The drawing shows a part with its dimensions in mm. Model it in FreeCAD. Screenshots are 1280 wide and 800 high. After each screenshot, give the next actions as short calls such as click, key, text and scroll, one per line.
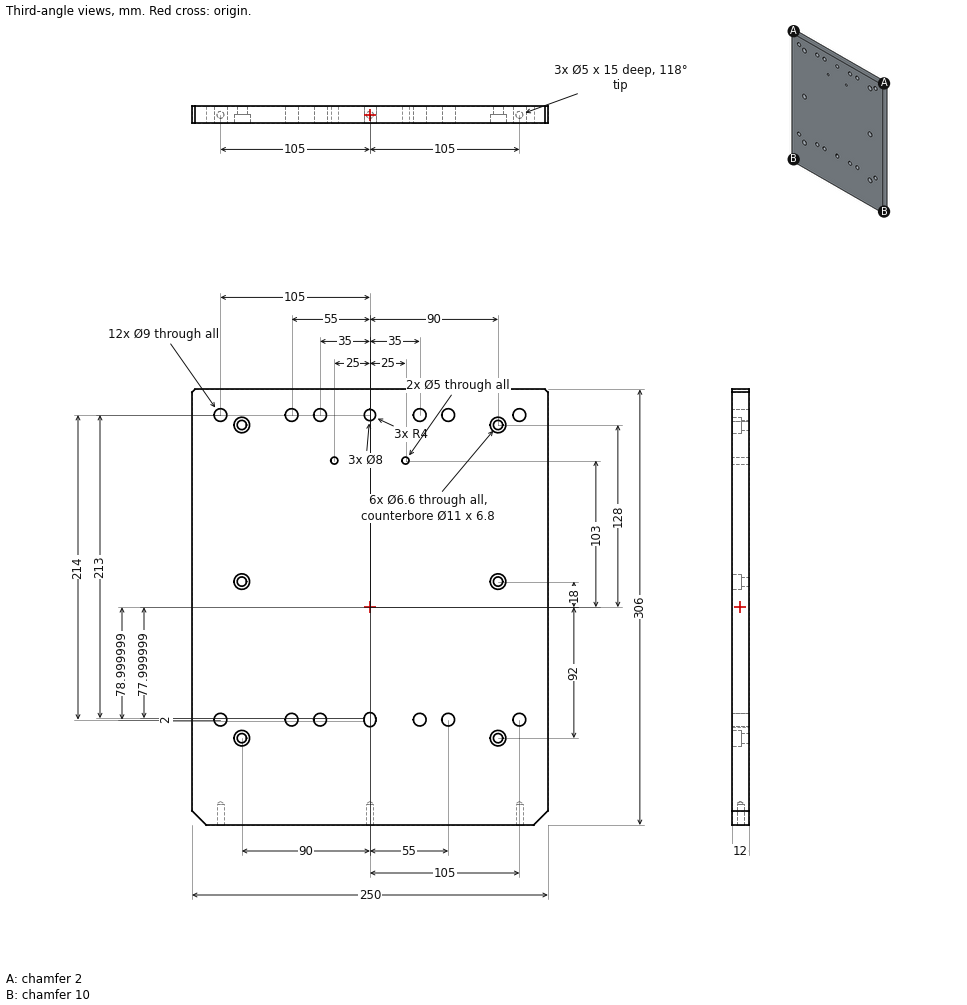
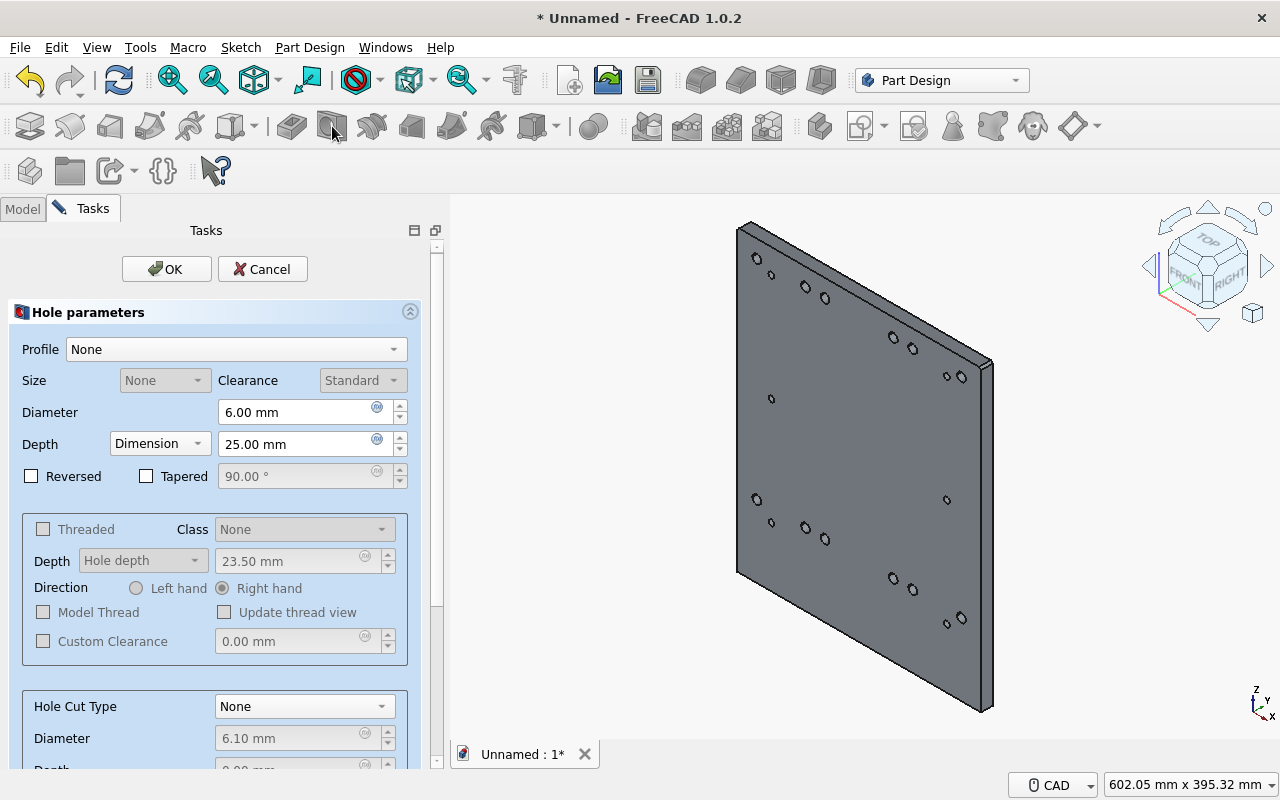
triple_click(305, 412)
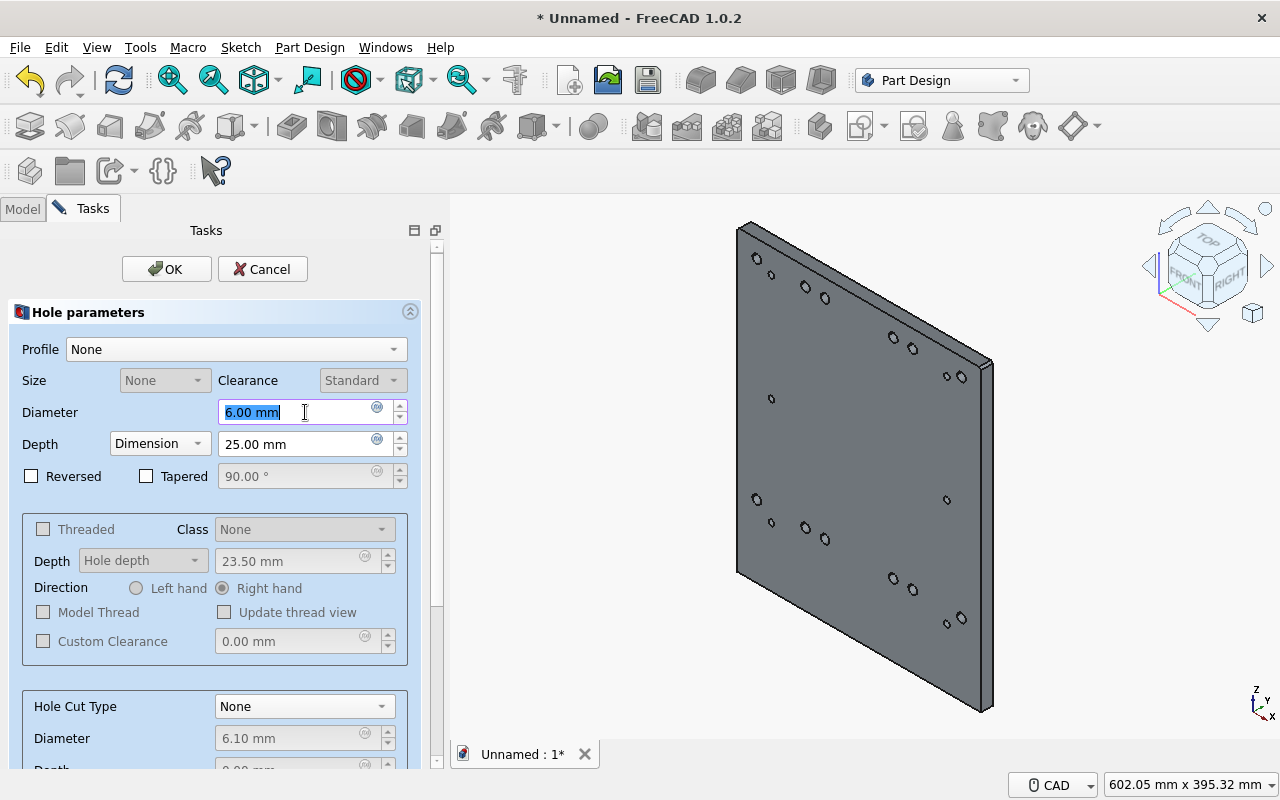
text(6.6)
key(Tab)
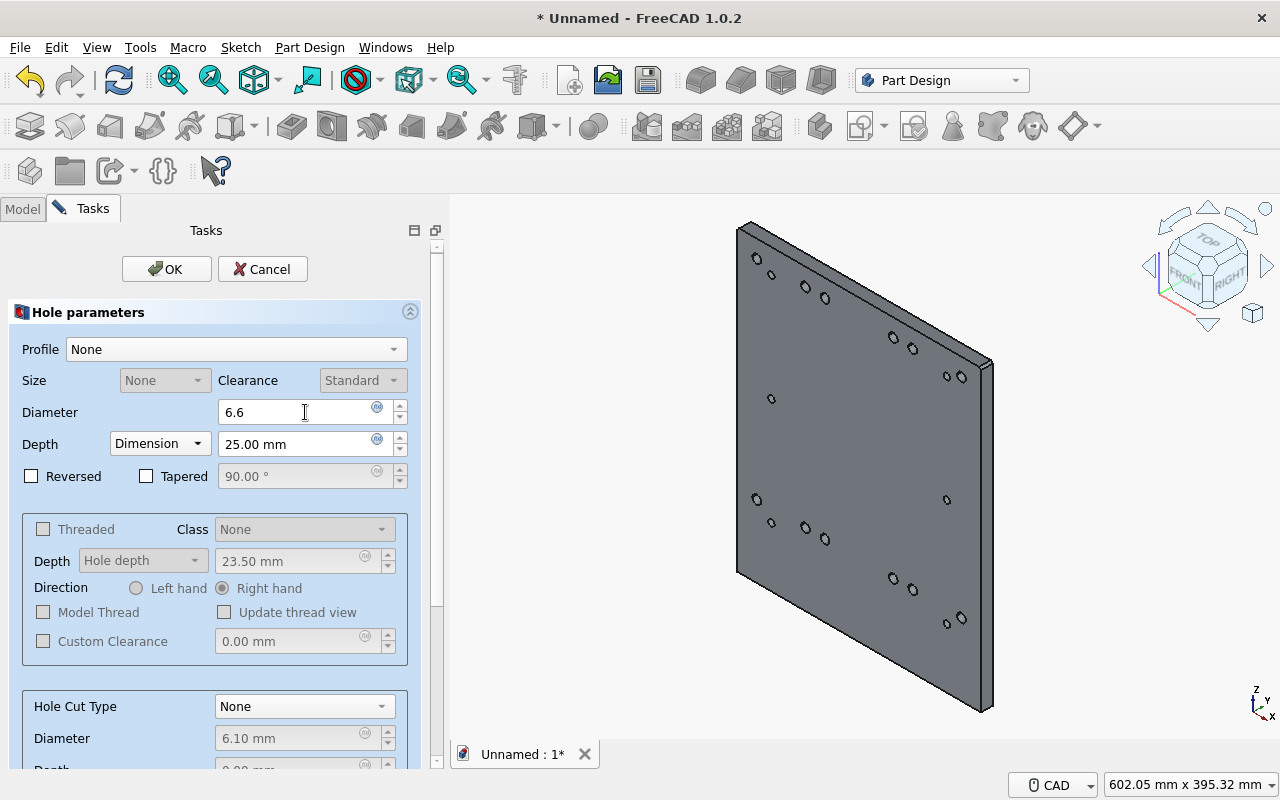
click(161, 444)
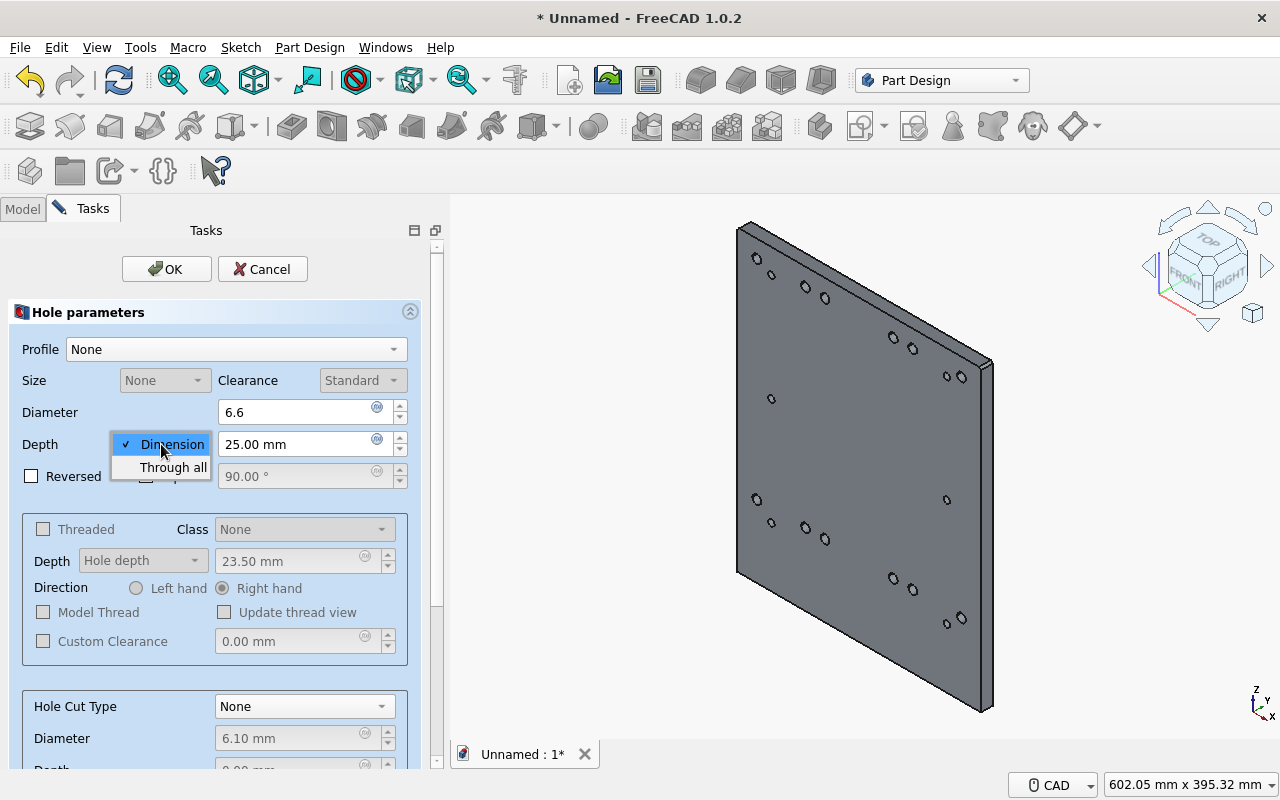
click(160, 468)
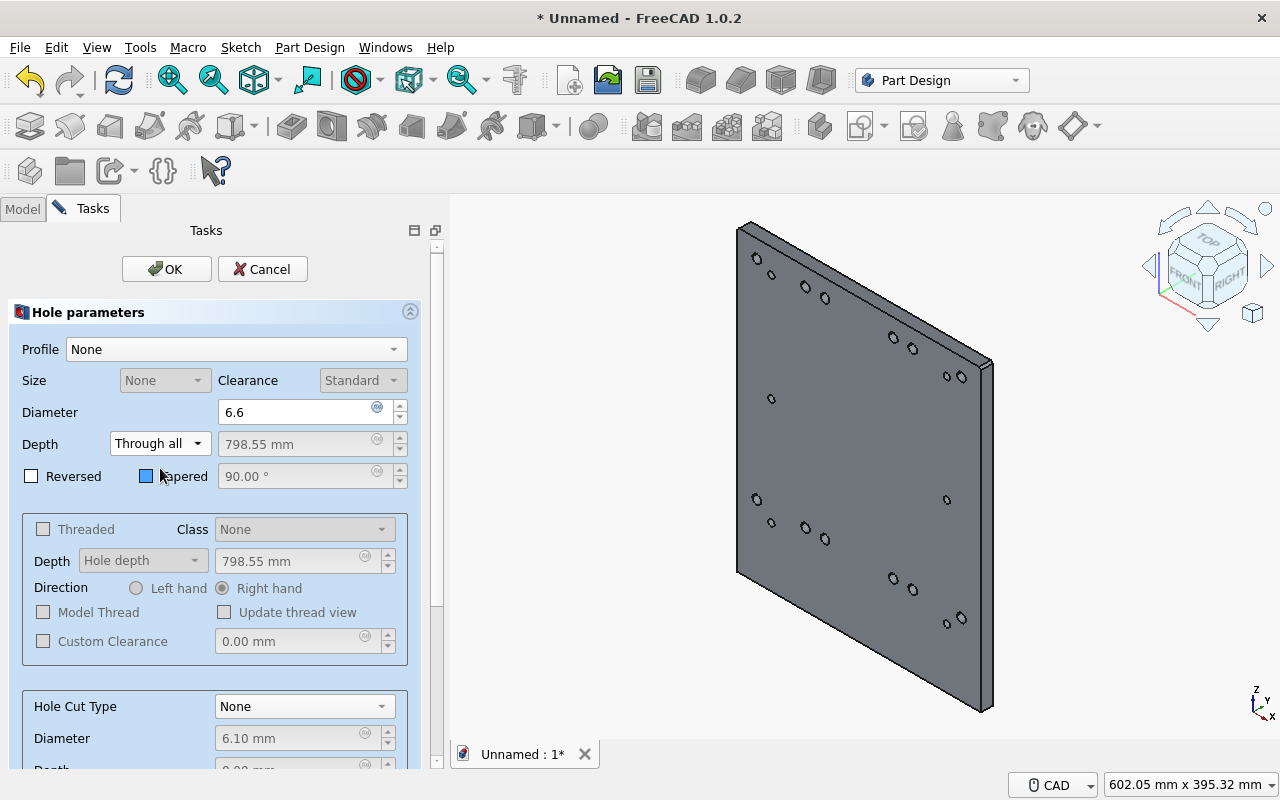
click(306, 706)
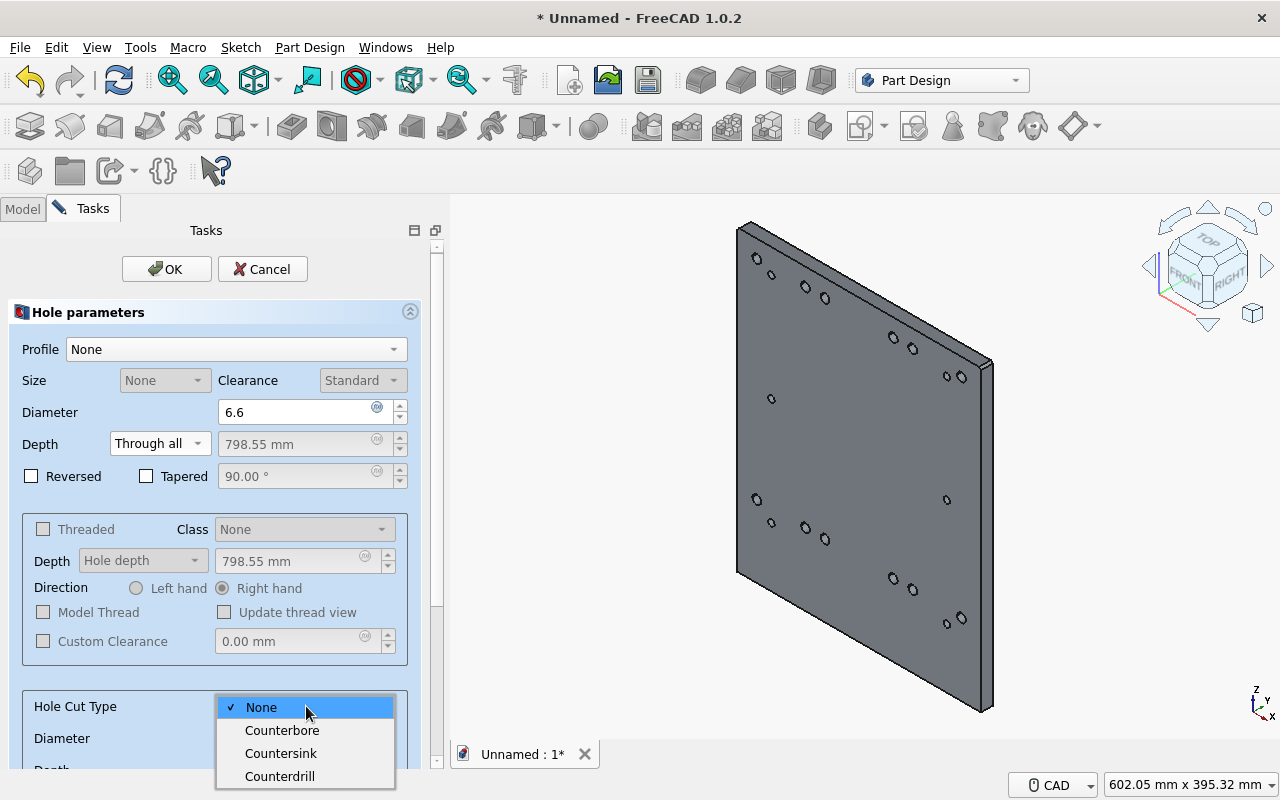
click(304, 730)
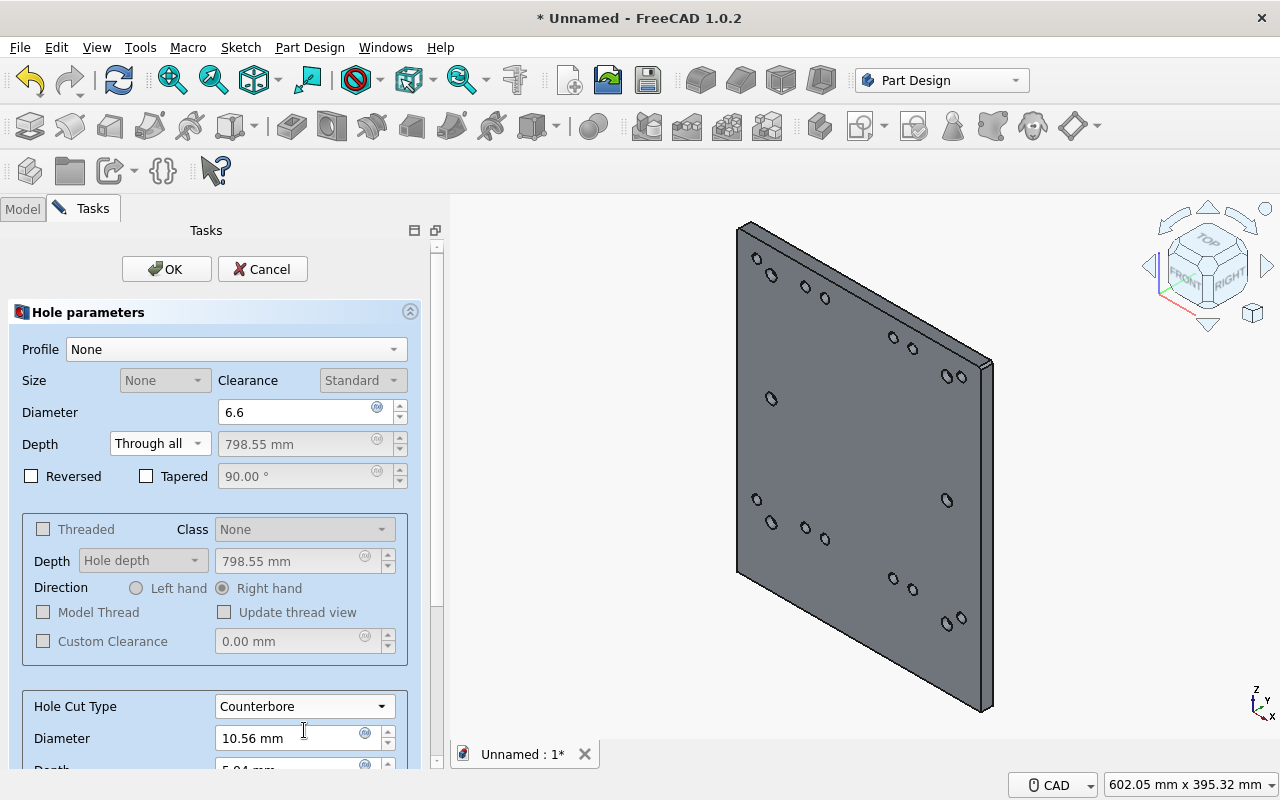
triple_click(298, 738)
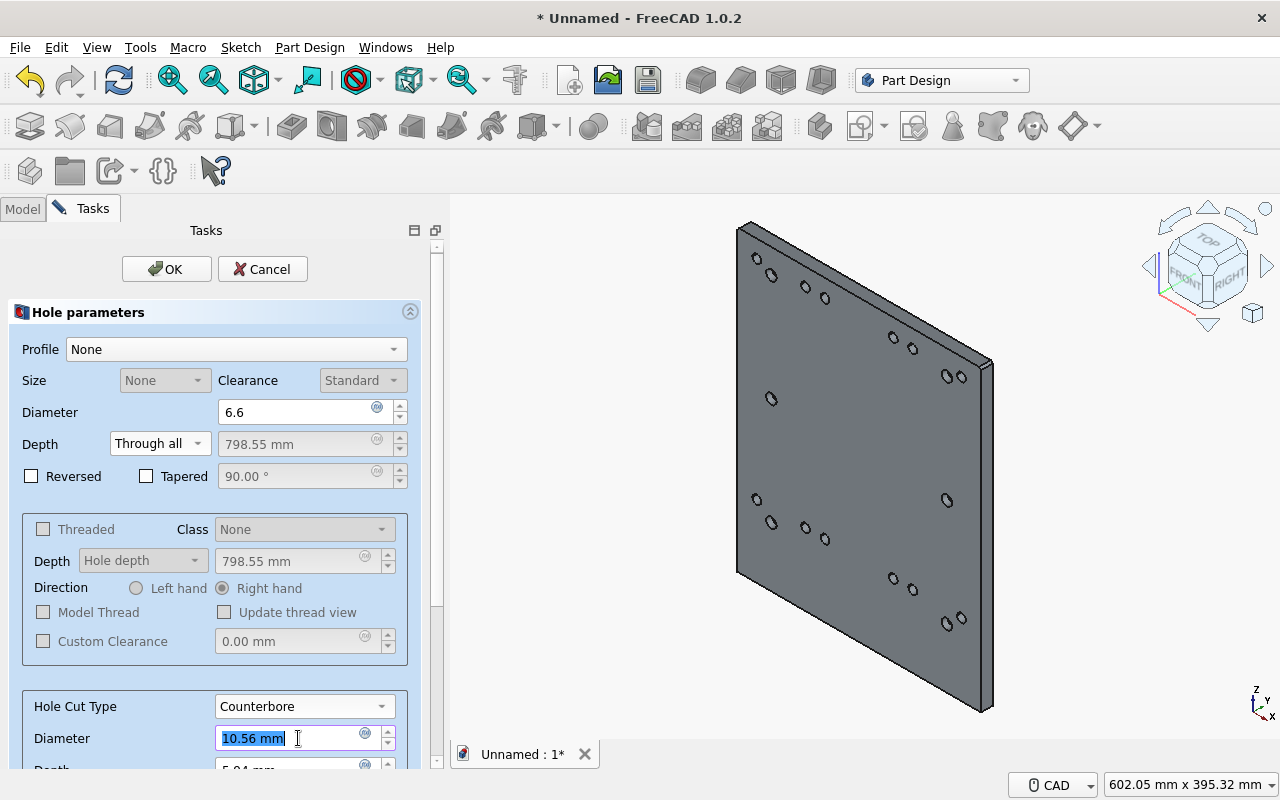
text(11)
key(Tab)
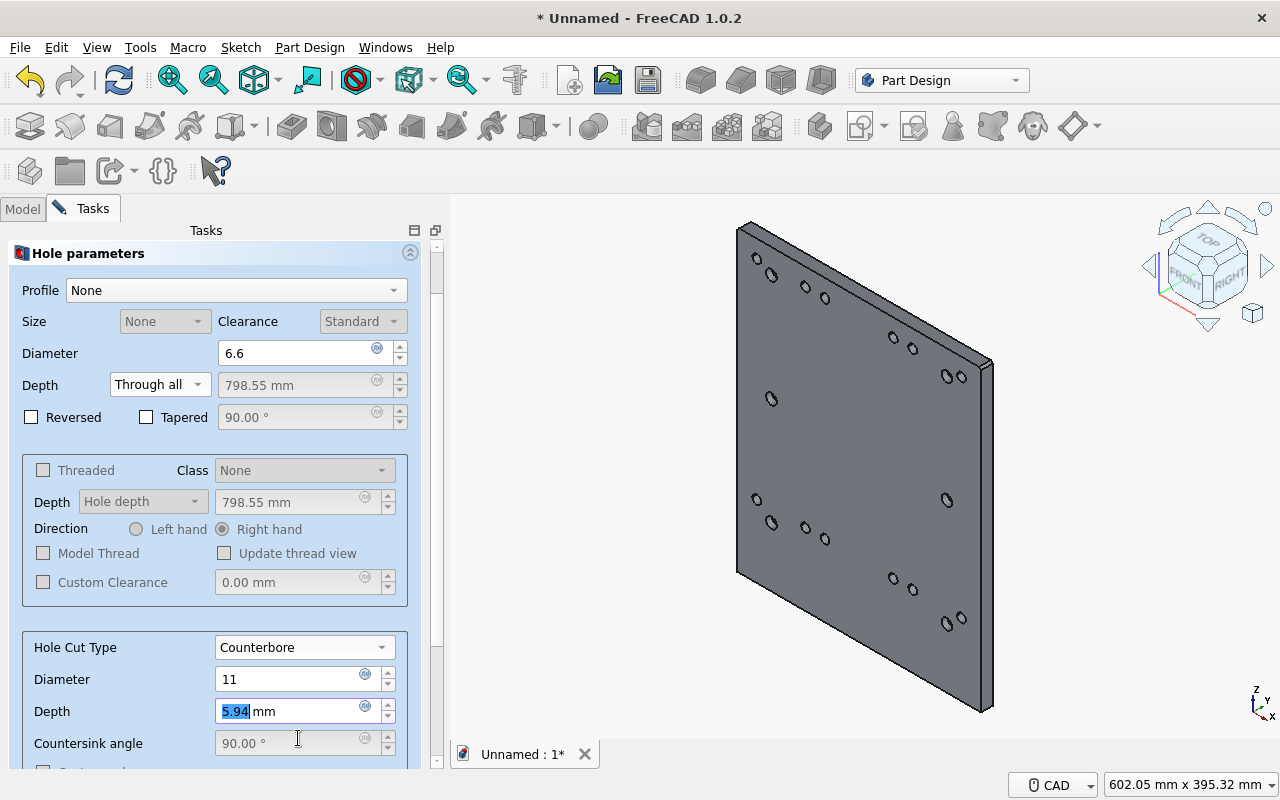
text(6.8)
key(Tab)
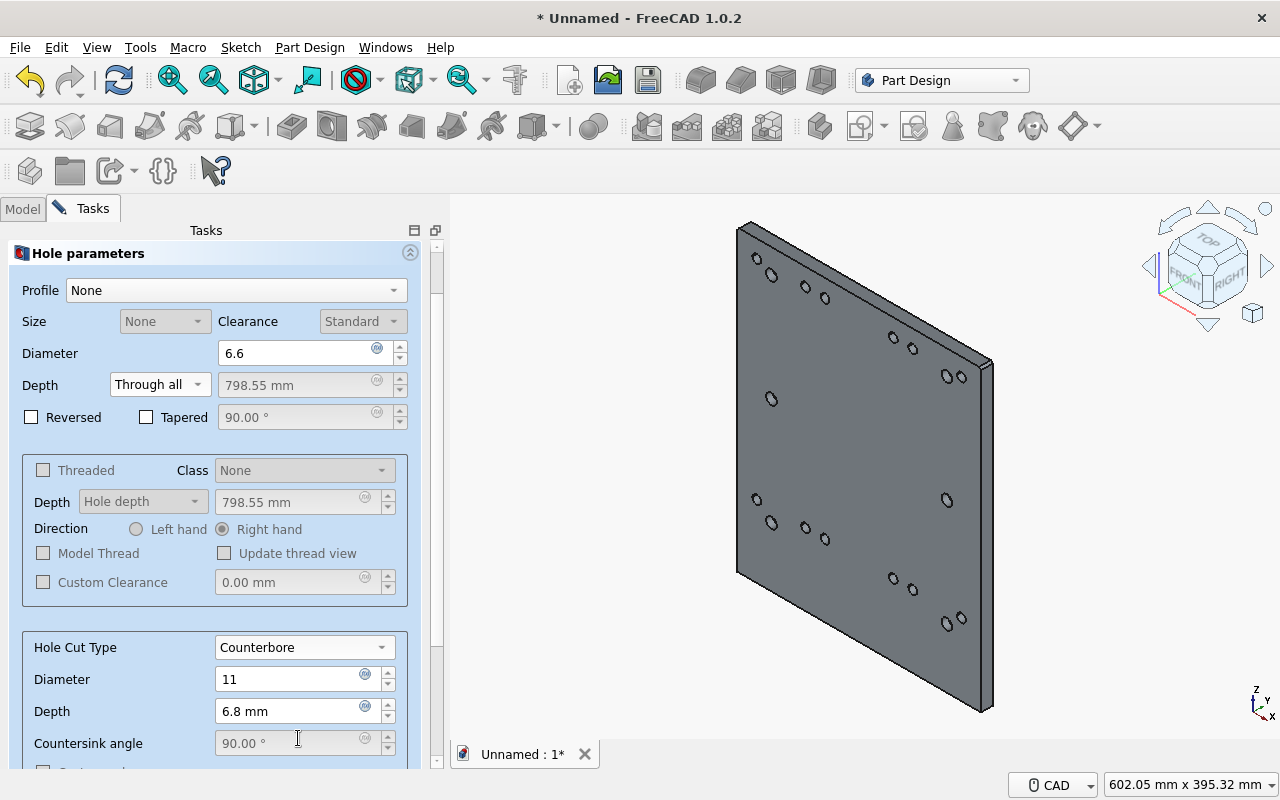
scroll(437, 504, up, 2)